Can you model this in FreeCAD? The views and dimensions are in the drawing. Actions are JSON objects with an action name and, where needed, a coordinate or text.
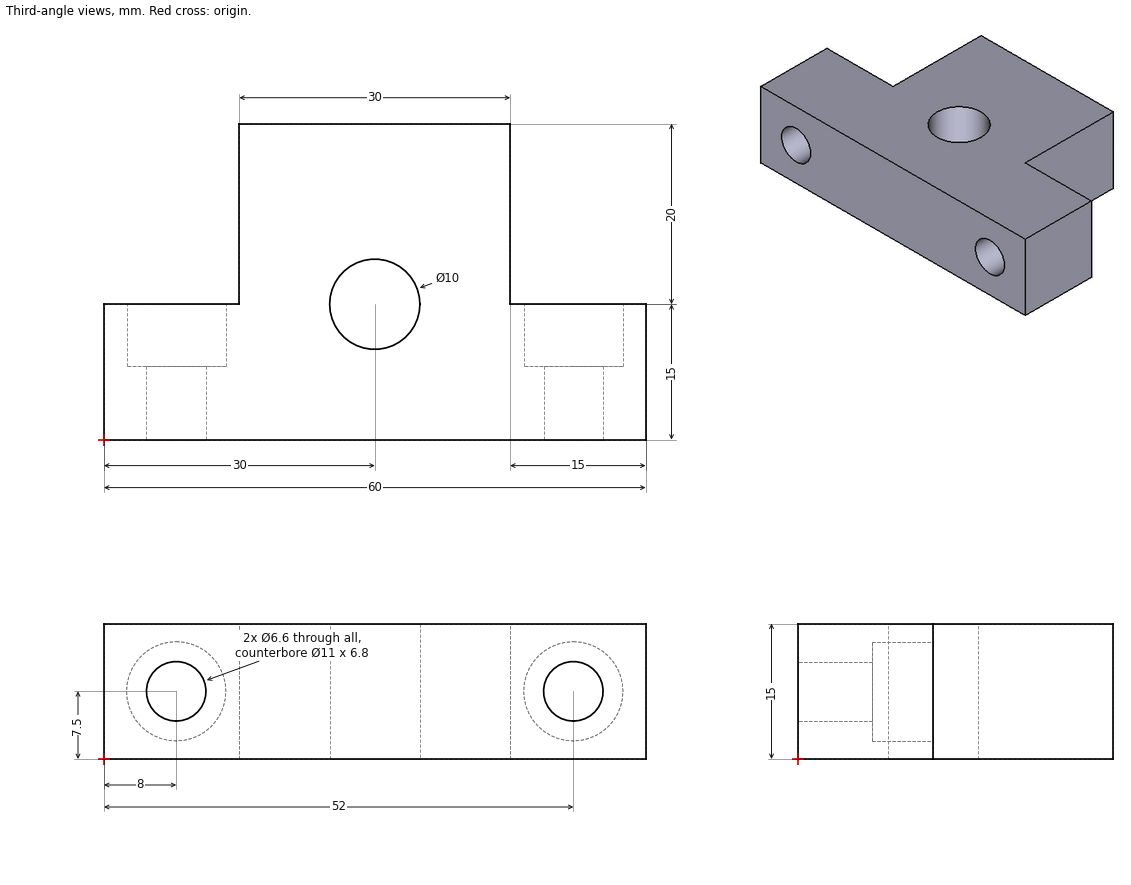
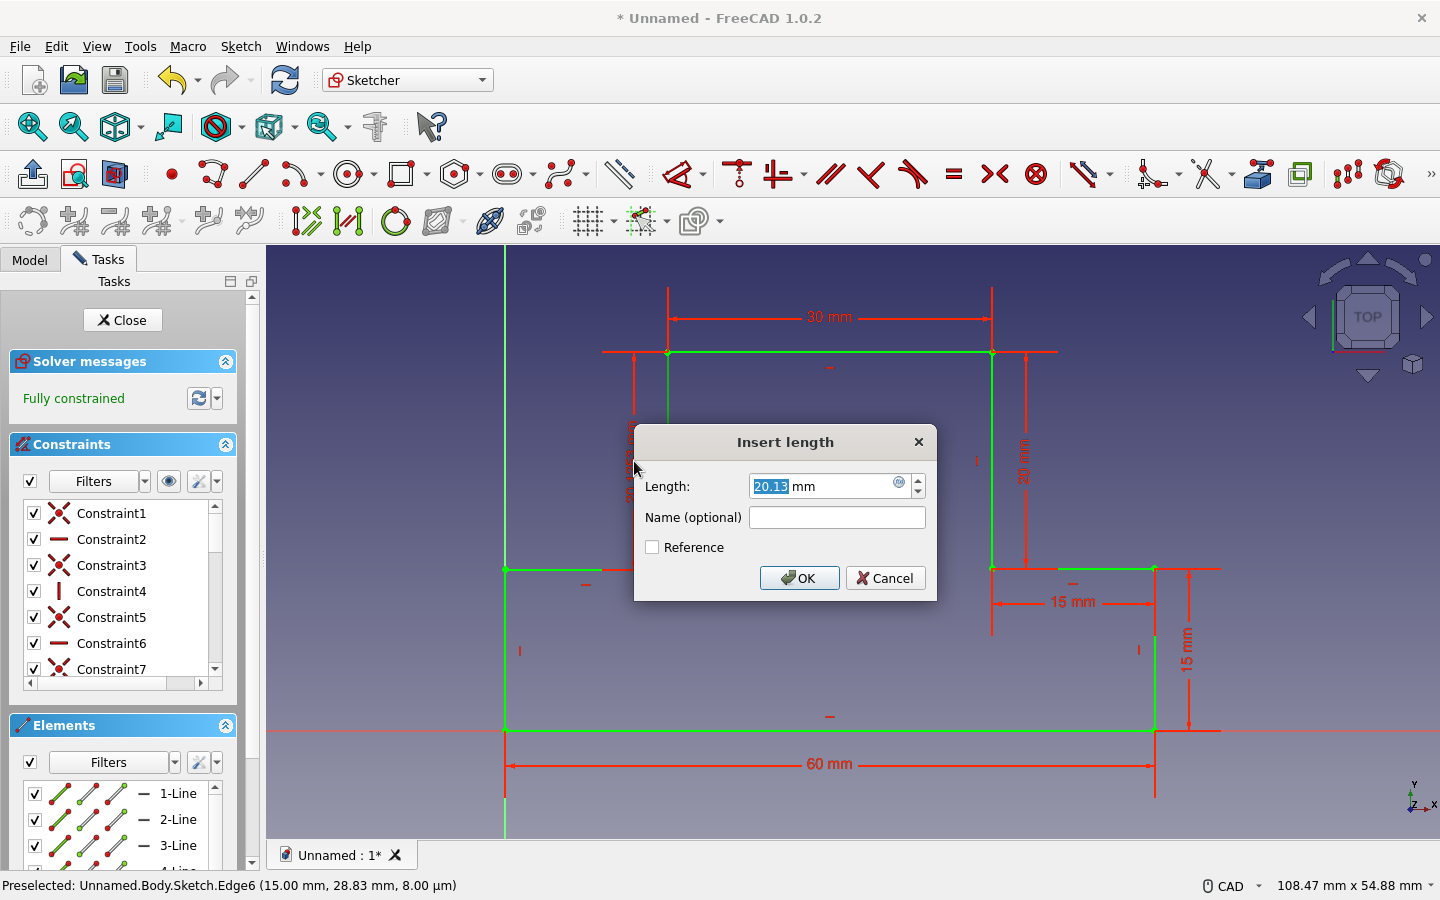
{"action": "type", "text": "20"}
{"action": "key", "text": "Return"}
{"action": "key", "text": "Escape"}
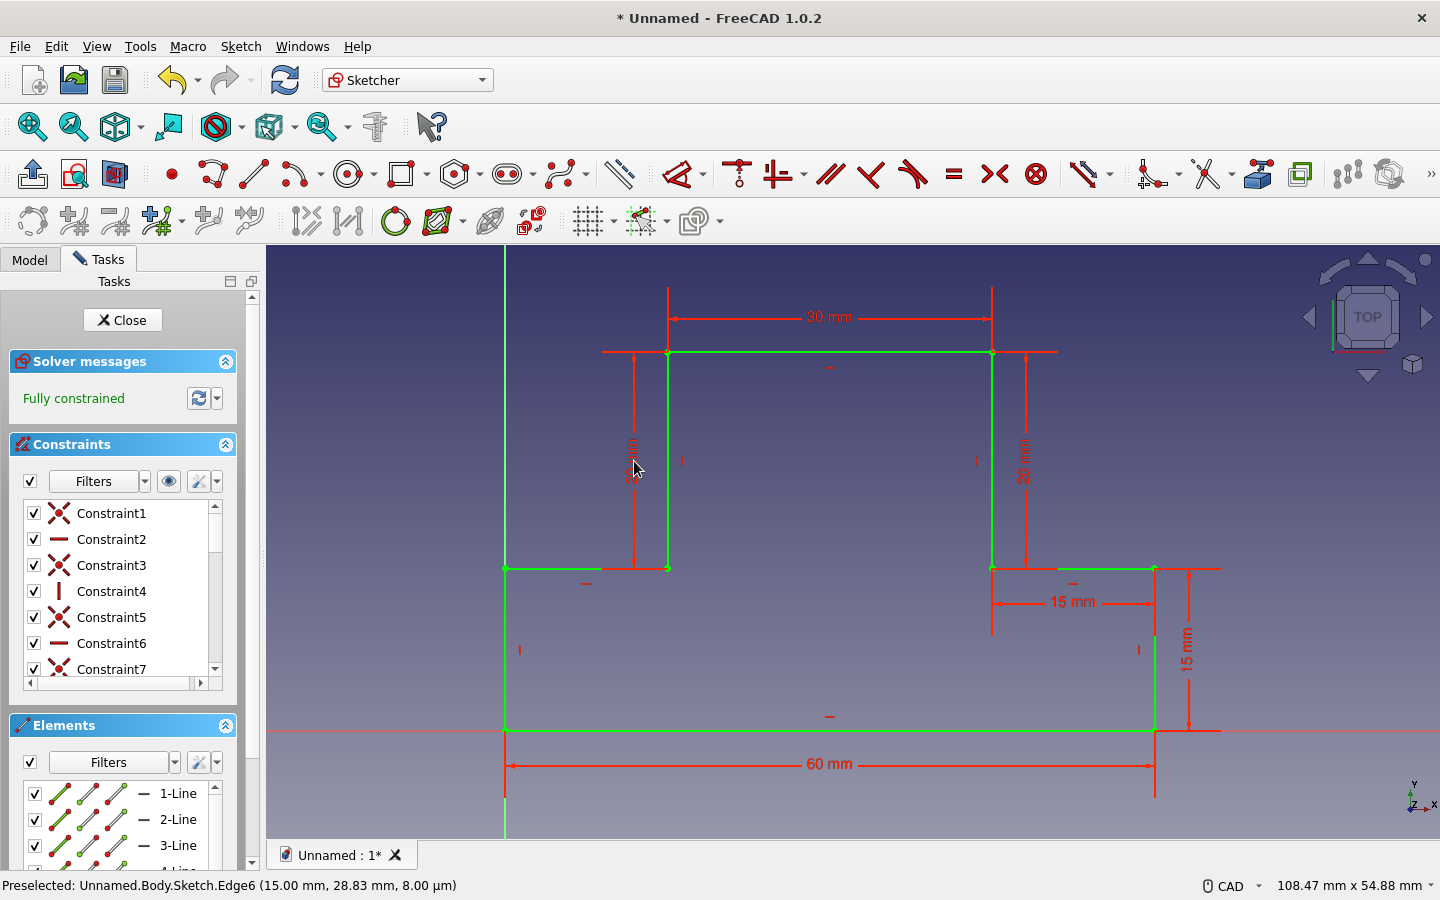
{"action": "left_click", "coordinate": [123, 320]}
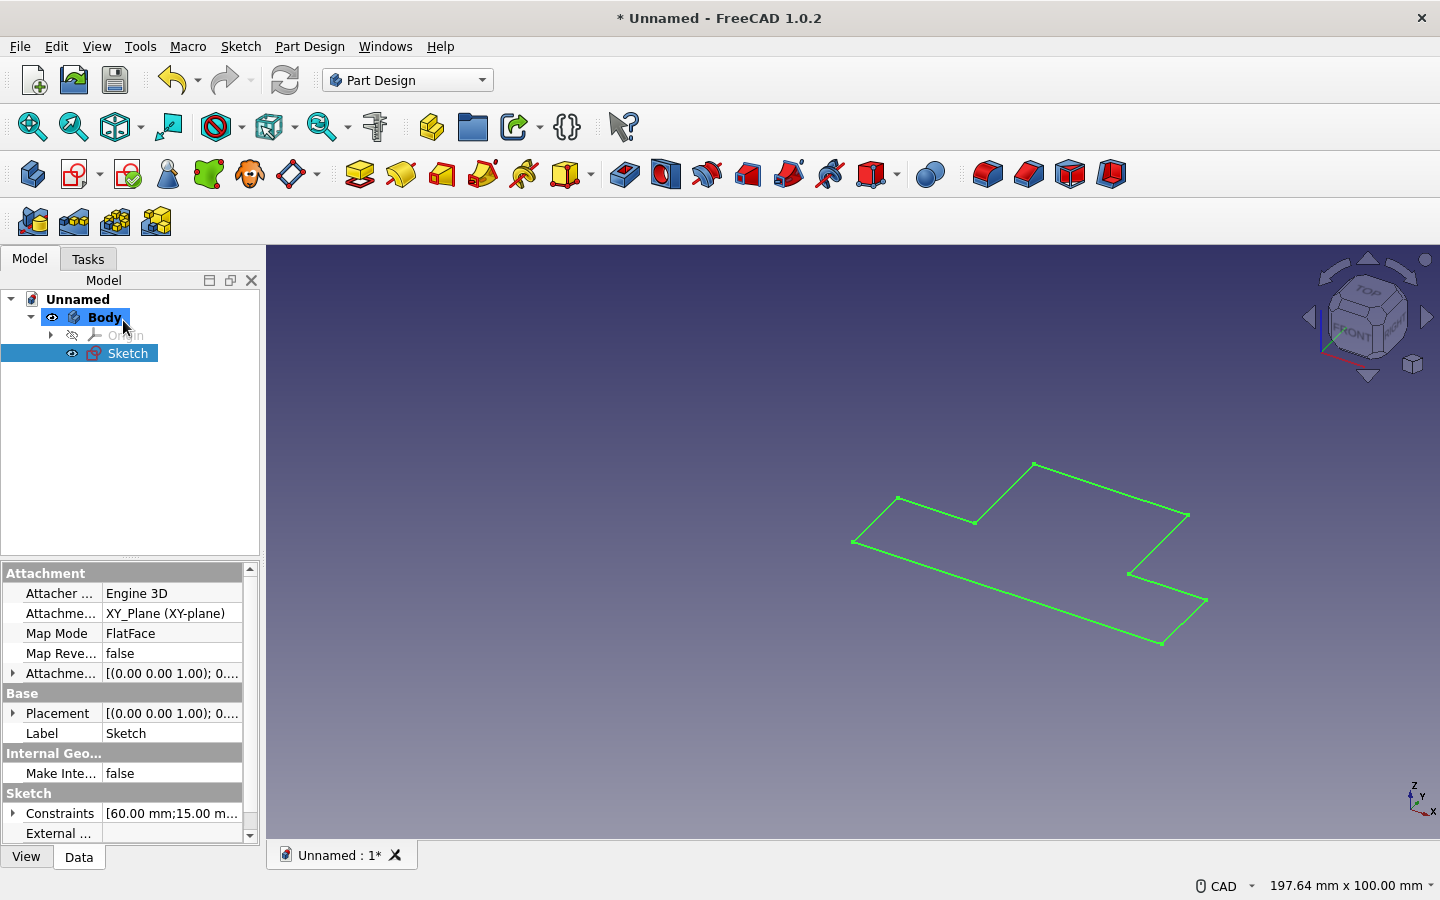
{"action": "left_click", "coordinate": [360, 174]}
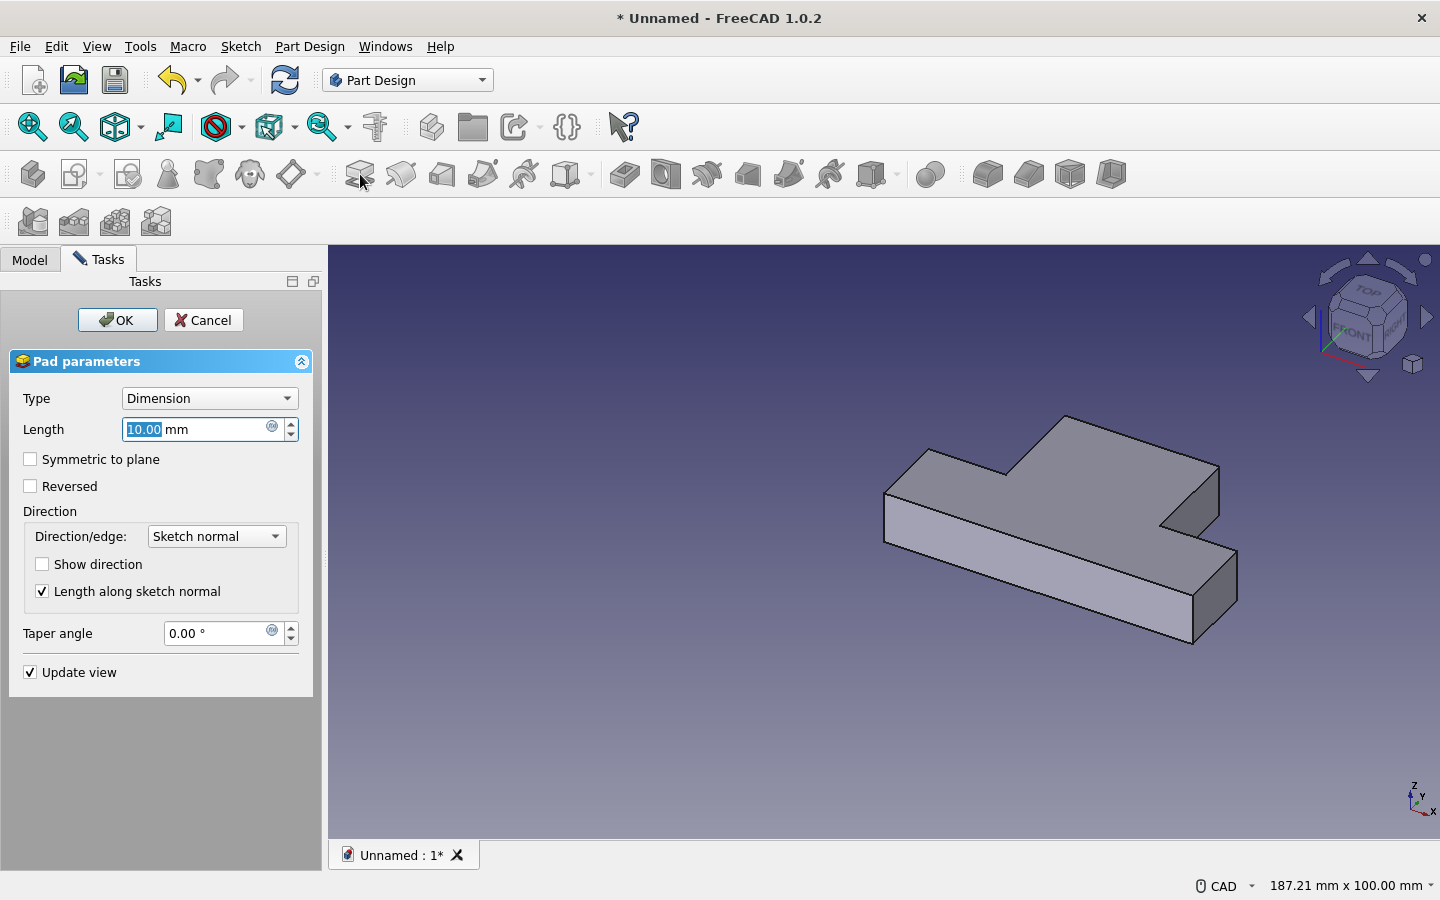
{"action": "type", "text": "15"}
{"action": "key", "text": "Tab"}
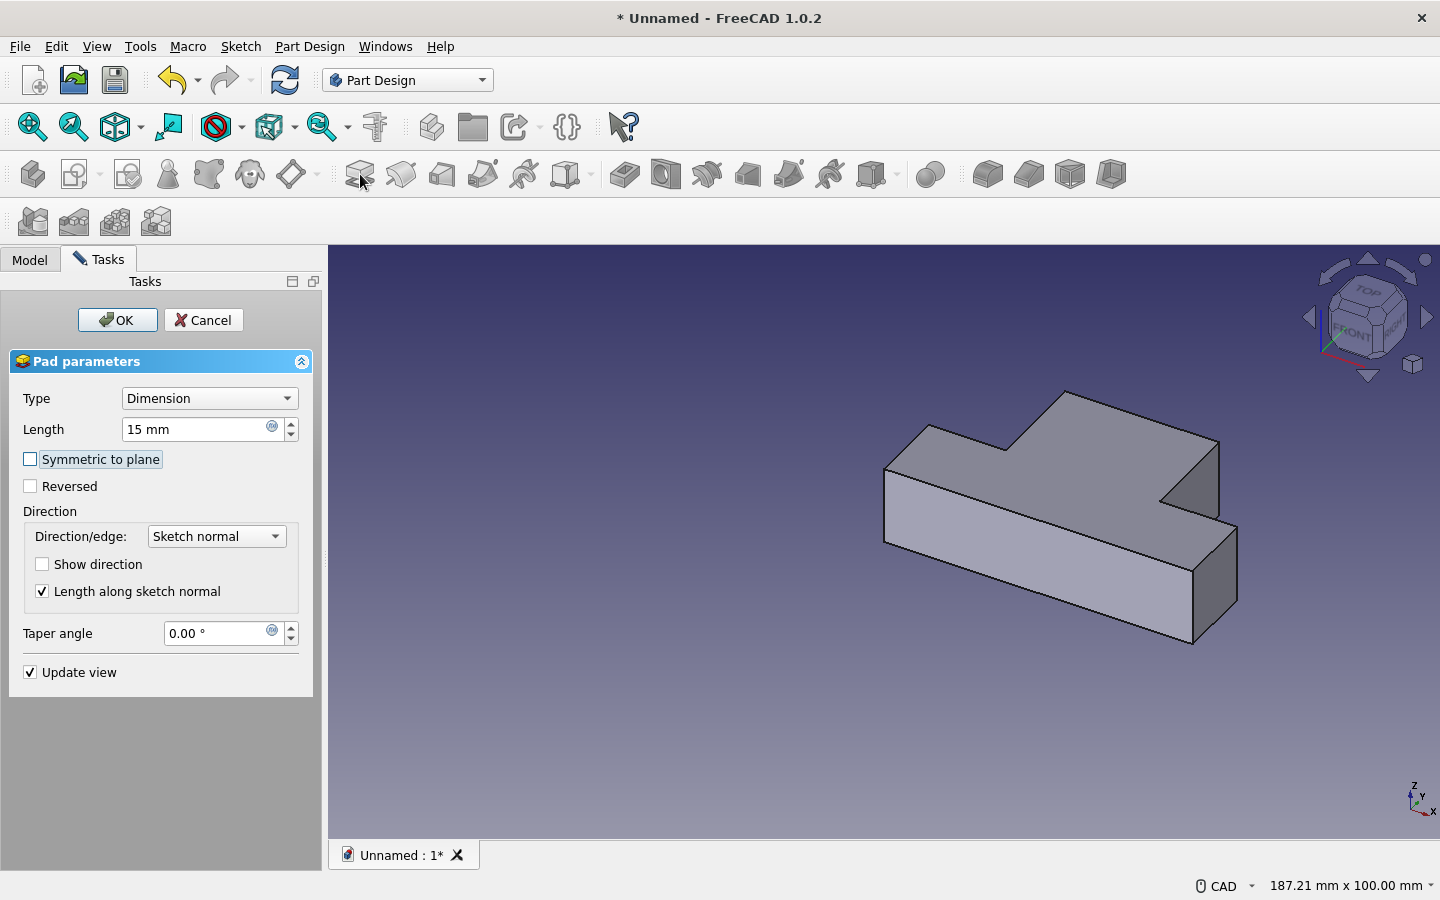
{"action": "left_click", "coordinate": [118, 320]}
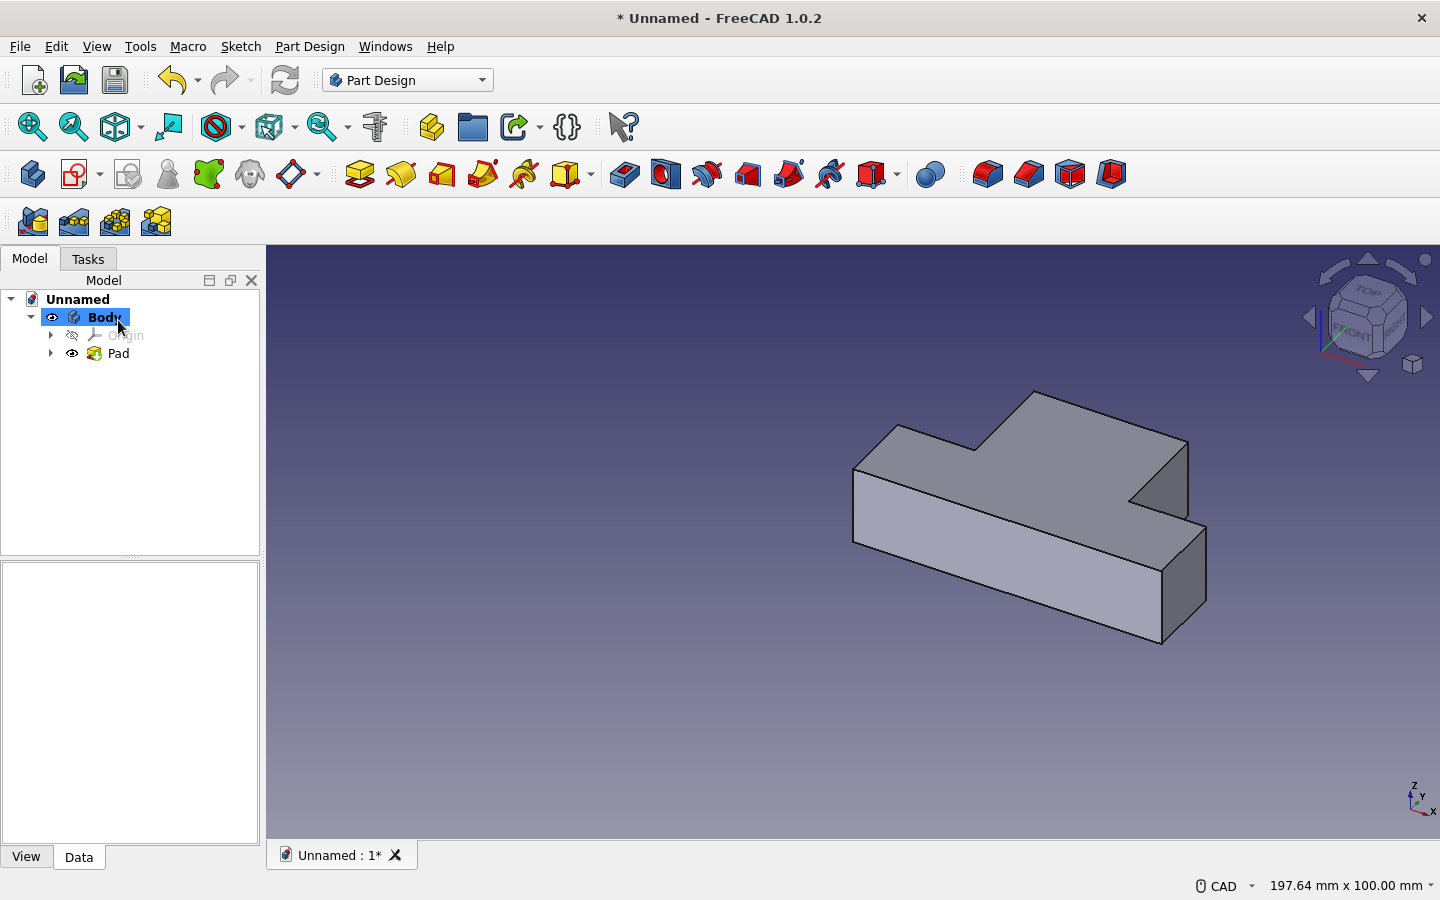
{"action": "left_click", "coordinate": [1059, 467]}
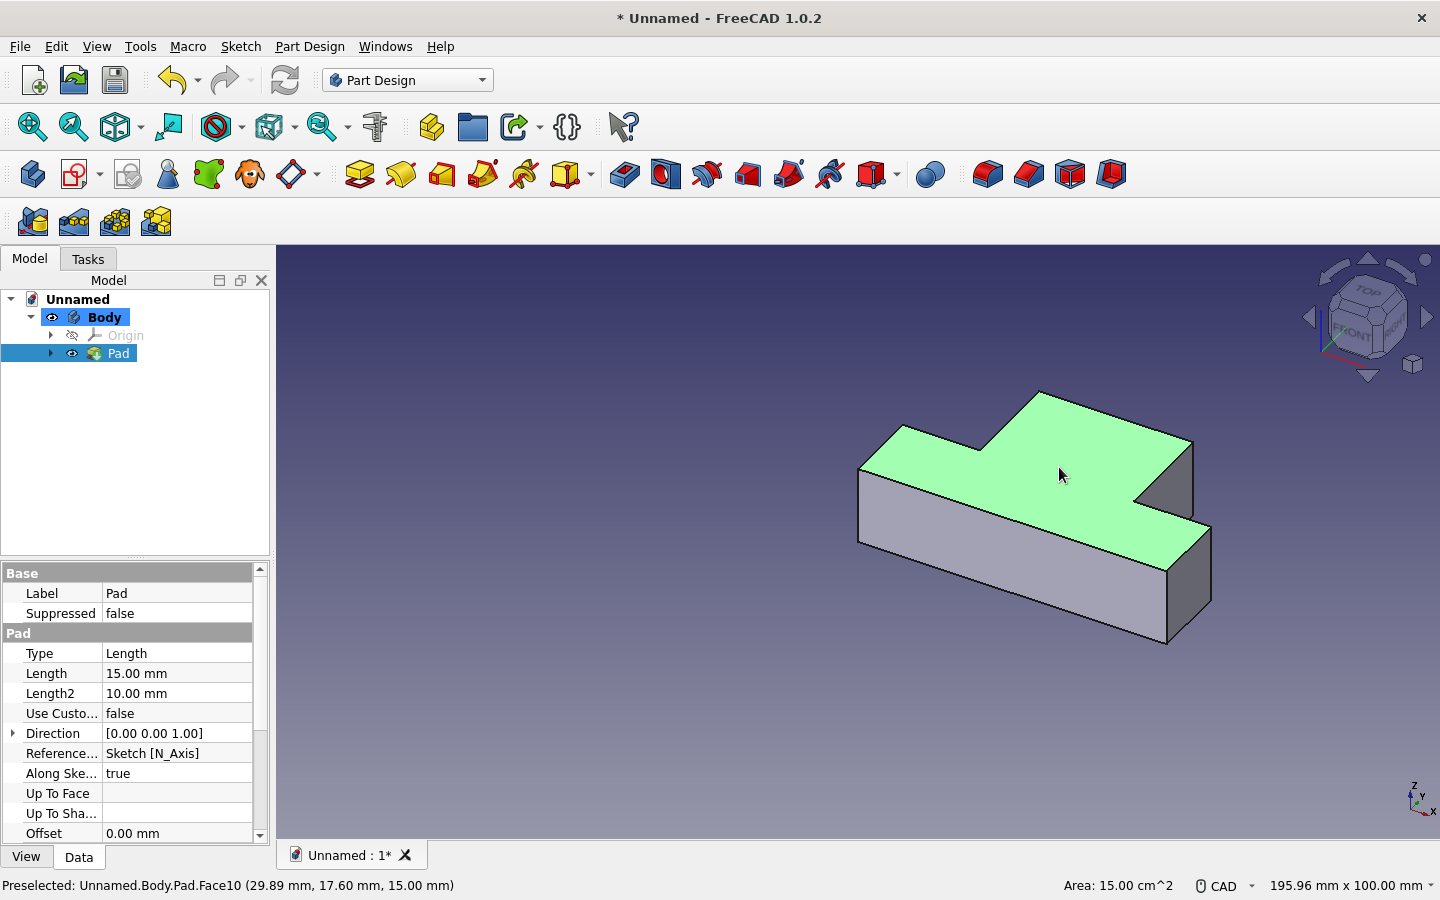
{"action": "left_click", "coordinate": [74, 174]}